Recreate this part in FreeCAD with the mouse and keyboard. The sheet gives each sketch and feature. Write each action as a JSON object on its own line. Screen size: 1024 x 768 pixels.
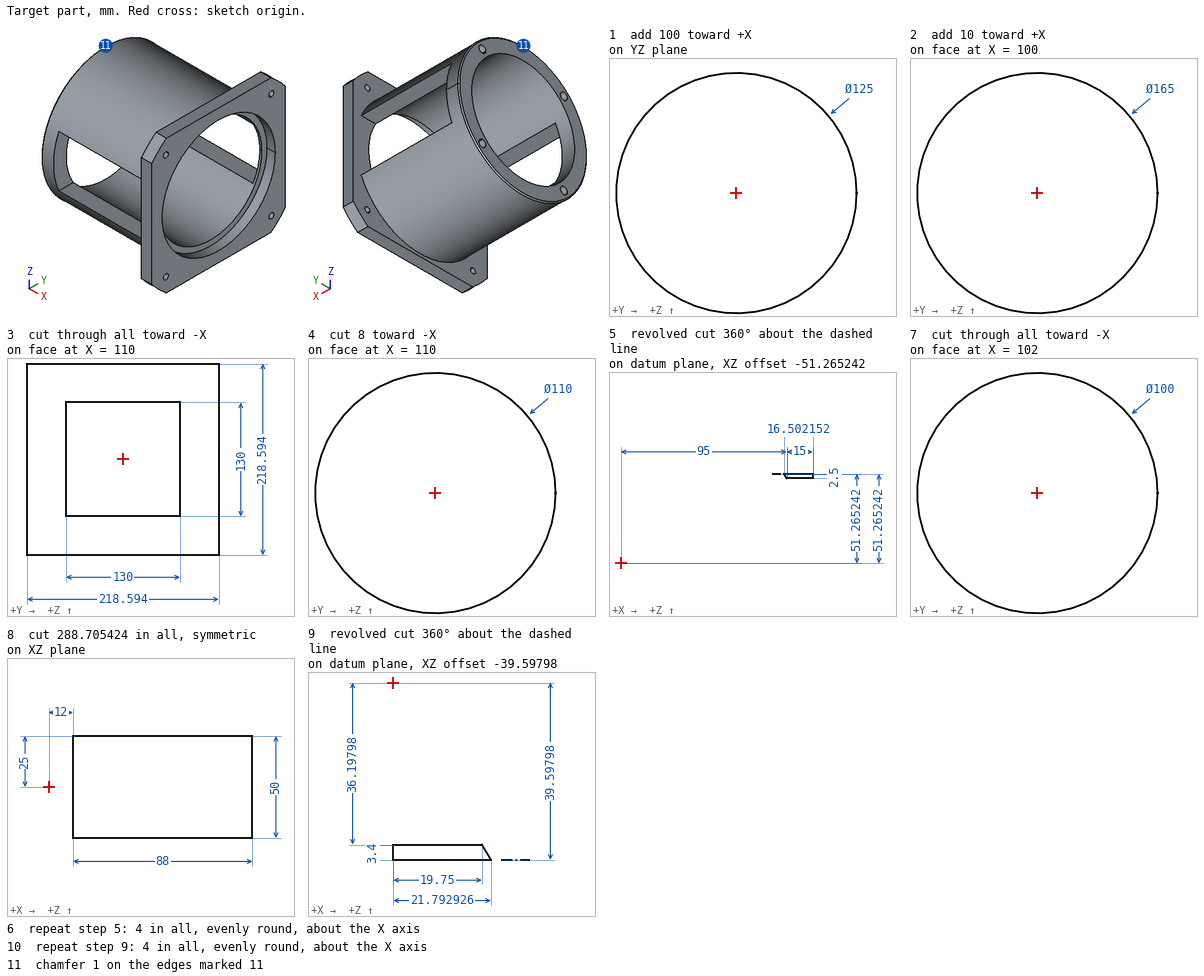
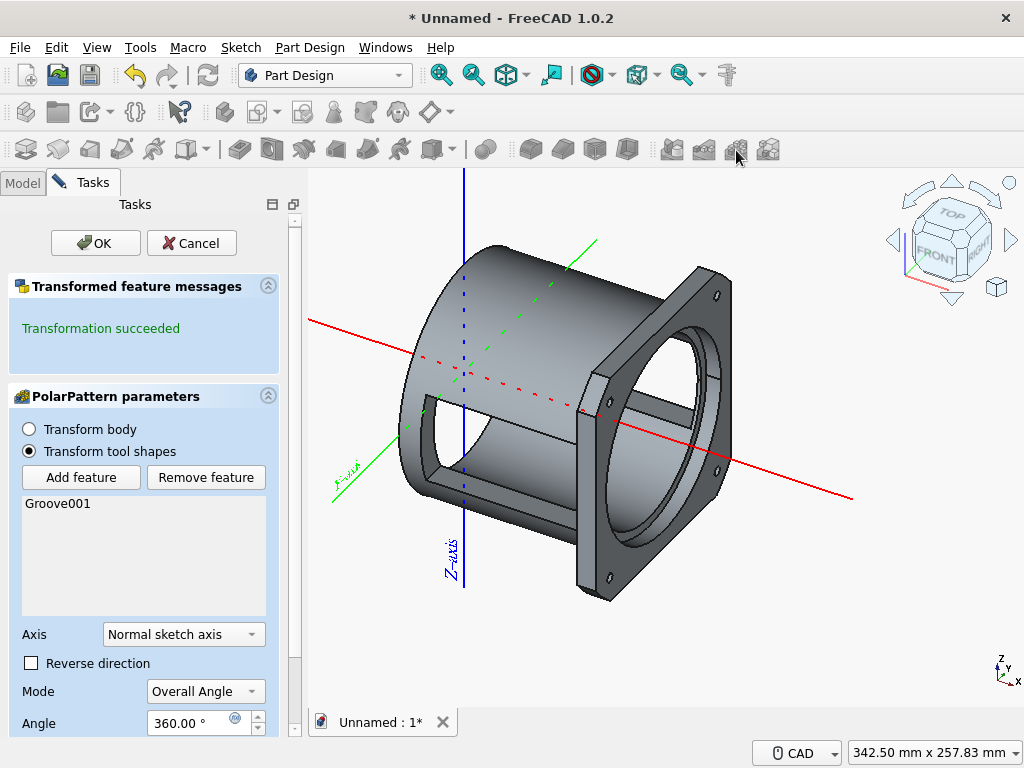
{"action": "left_click", "coordinate": [184, 634]}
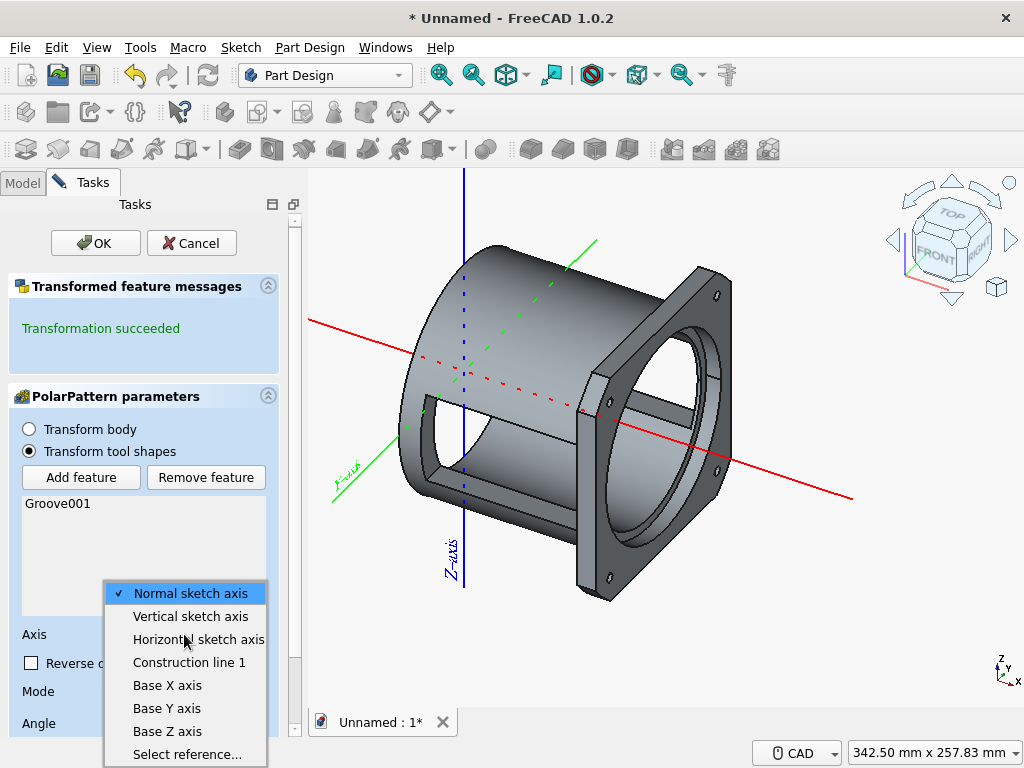
{"action": "left_click", "coordinate": [184, 686]}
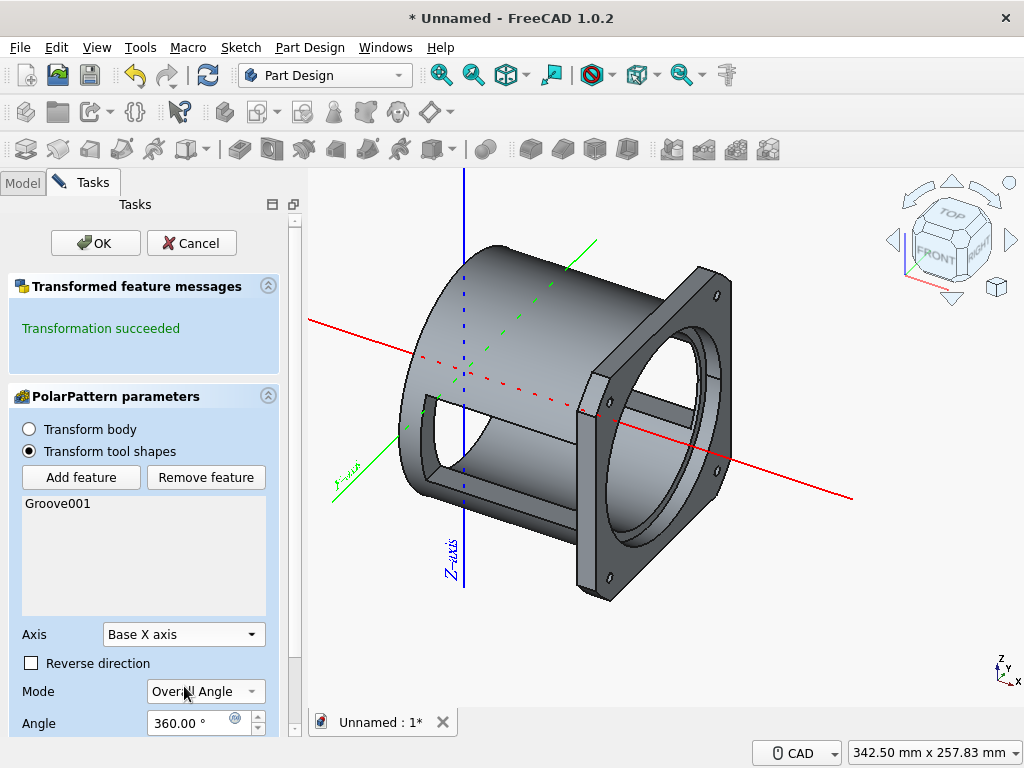
{"action": "scroll", "coordinate": [295, 475], "scroll_direction": "down", "scroll_amount": 2}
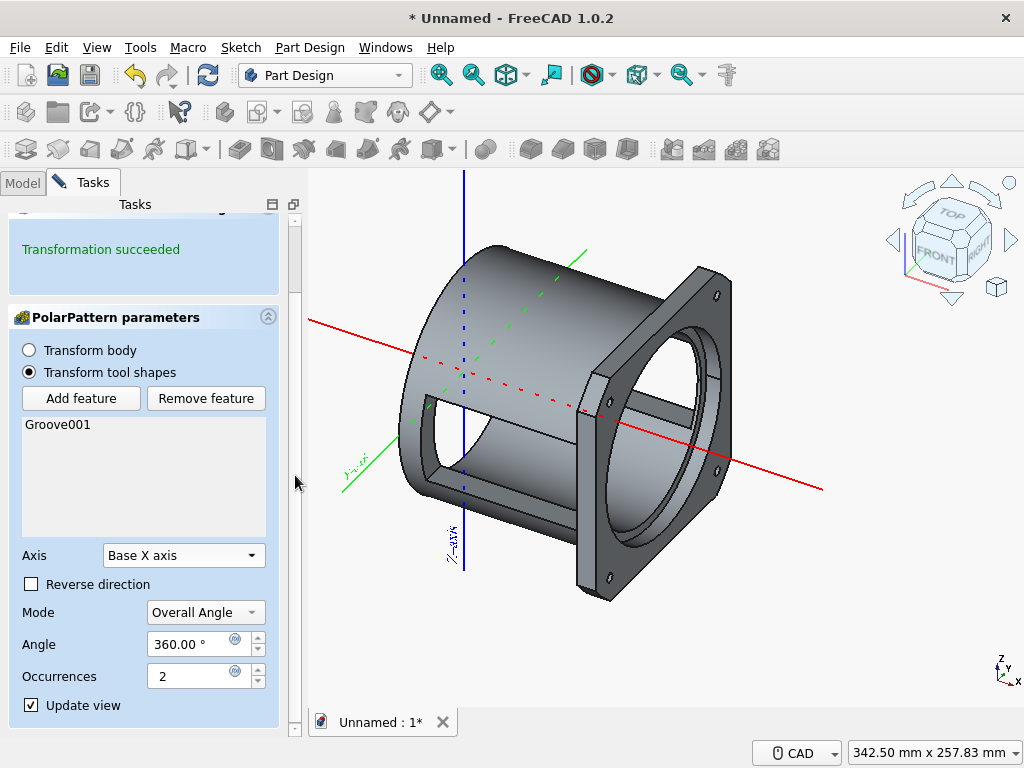
{"action": "triple_click", "coordinate": [198, 676]}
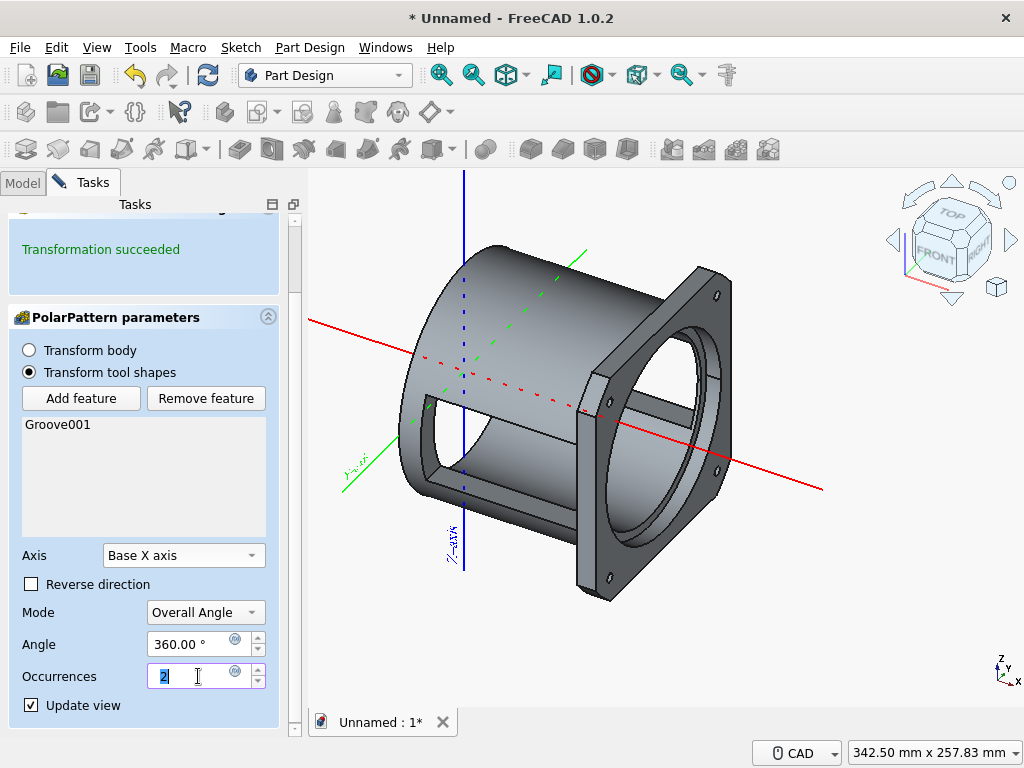
{"action": "type", "text": "4"}
{"action": "key", "text": "Tab"}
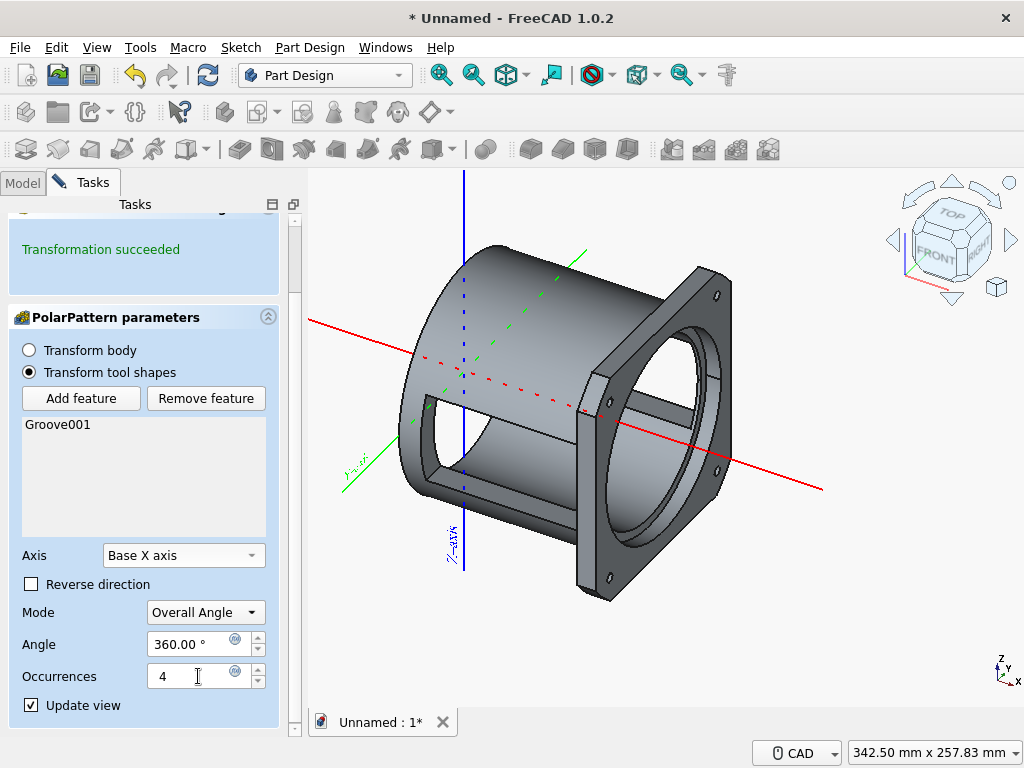
{"action": "scroll", "coordinate": [295, 475], "scroll_direction": "up", "scroll_amount": 3}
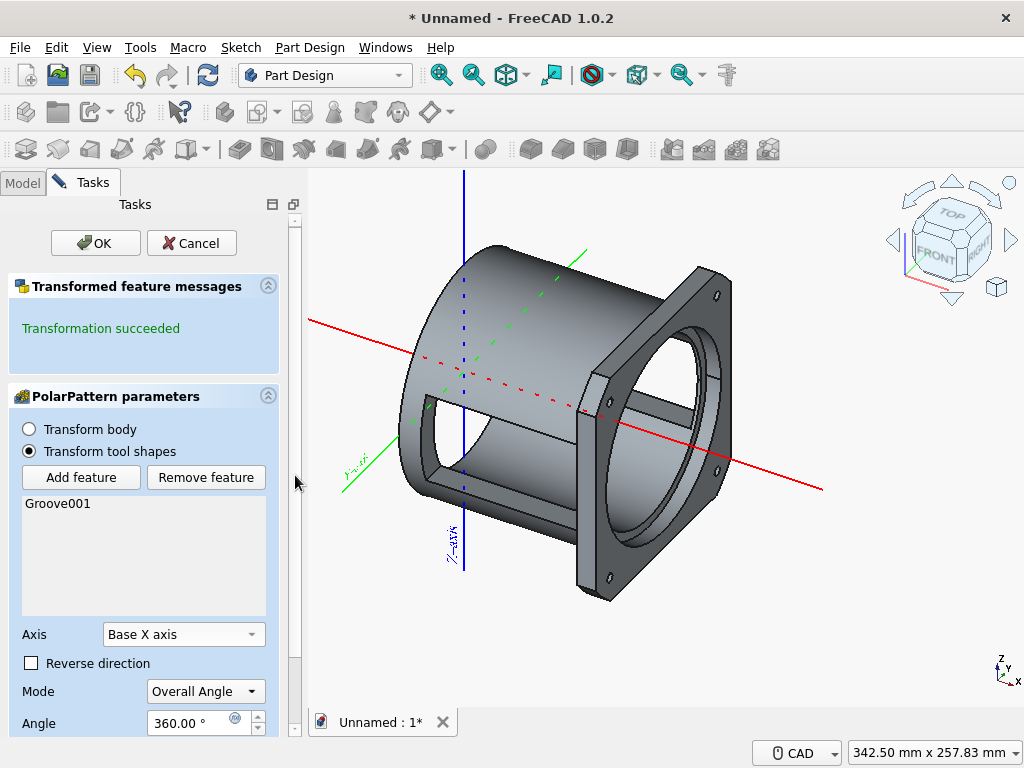
{"action": "left_click", "coordinate": [96, 243]}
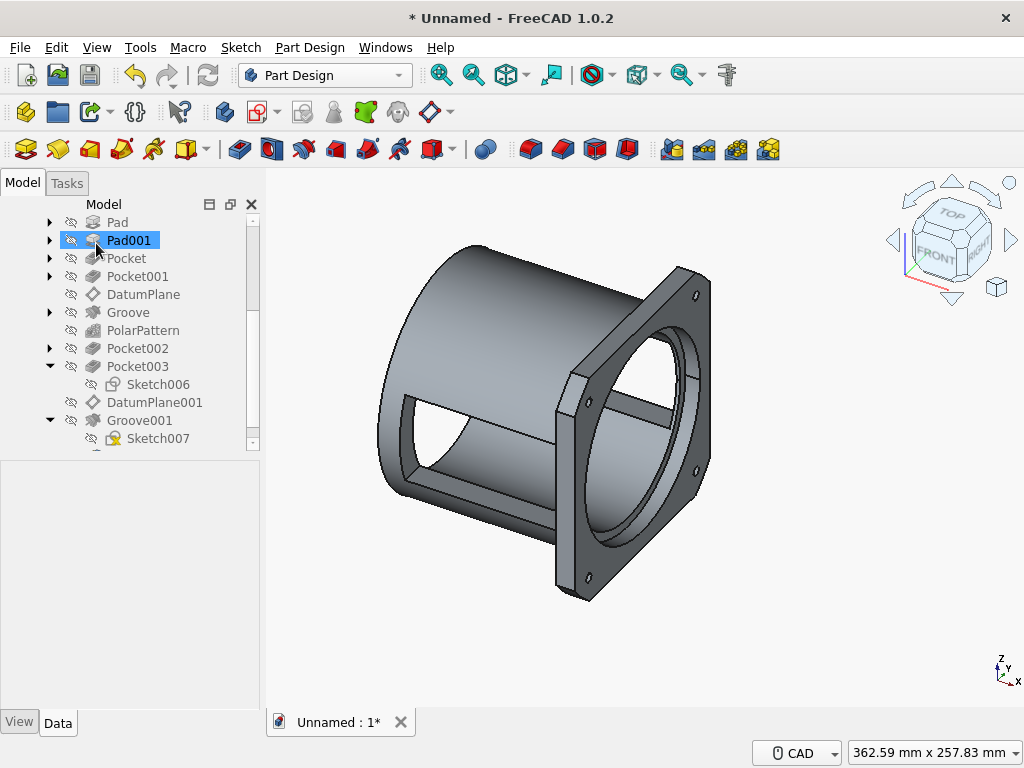
{"action": "key", "text": "0"}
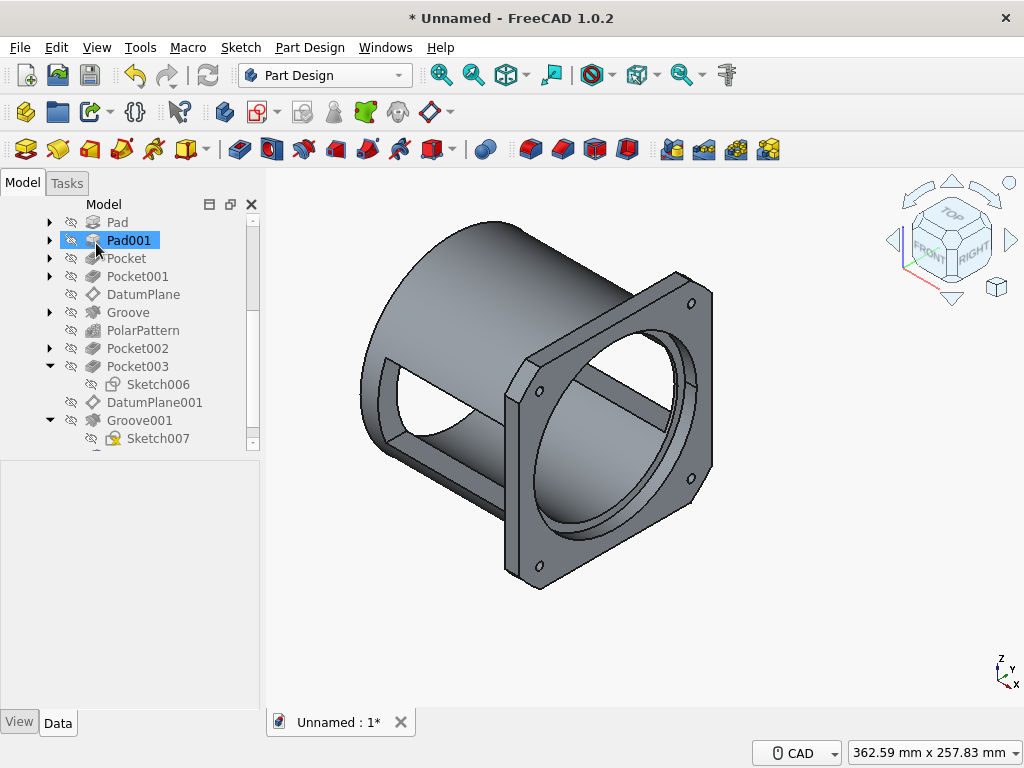
{"action": "key", "text": "2"}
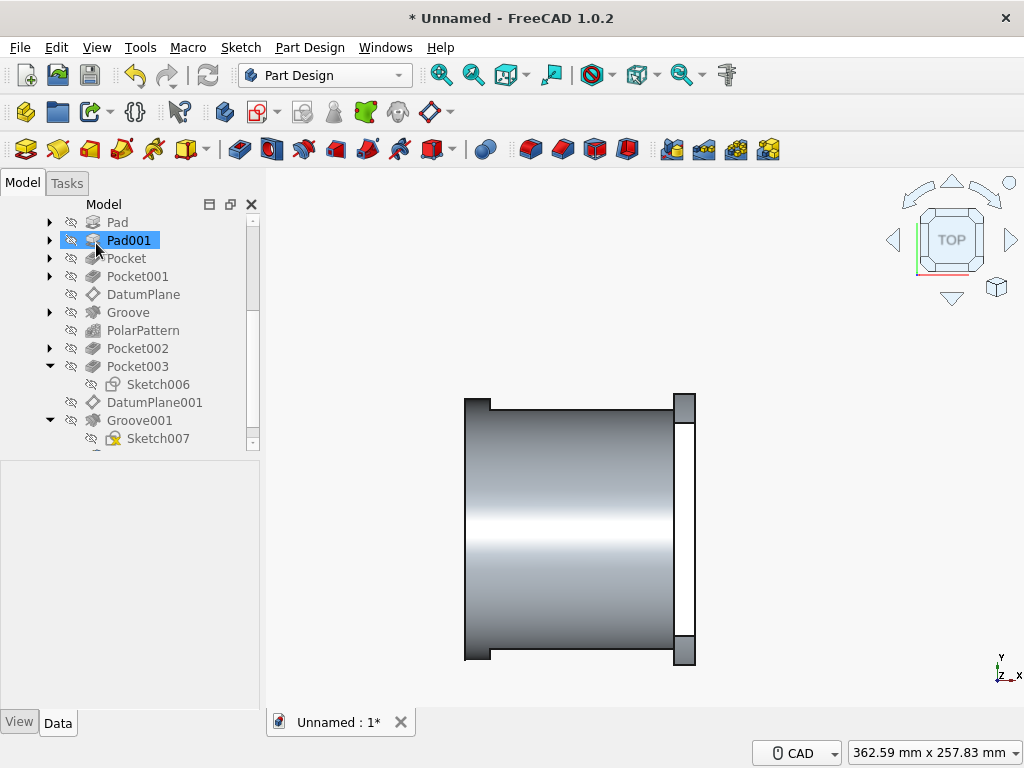
{"action": "key", "text": "1"}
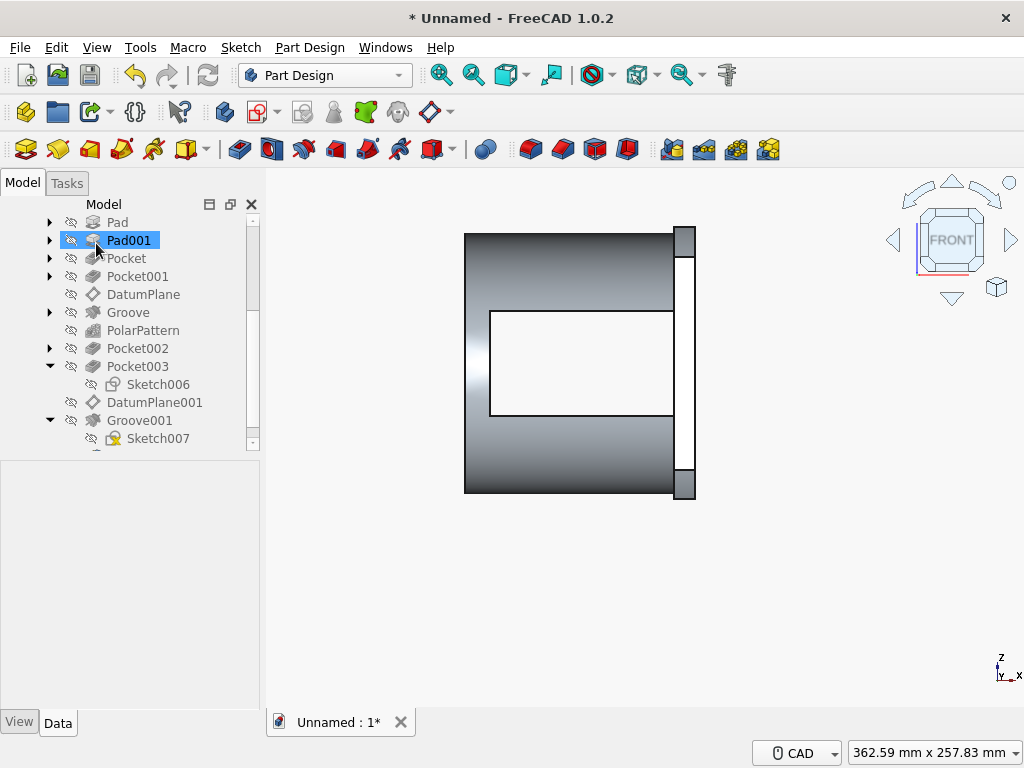
{"action": "left_click", "coordinate": [465, 362]}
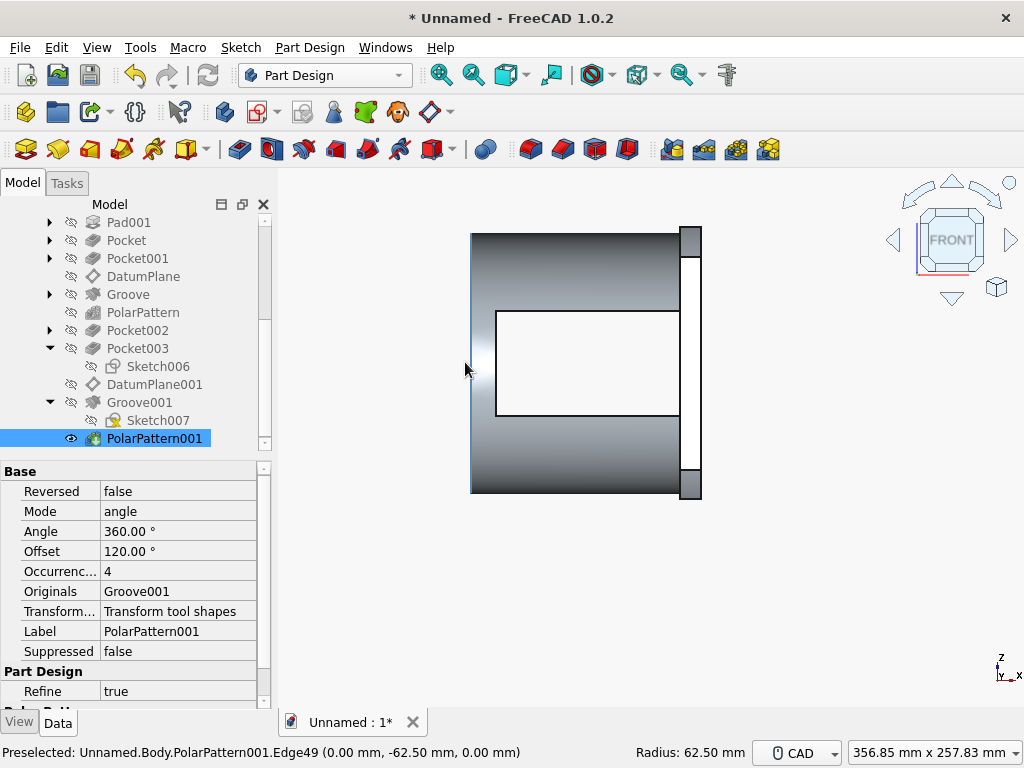
{"action": "left_click", "coordinate": [564, 150]}